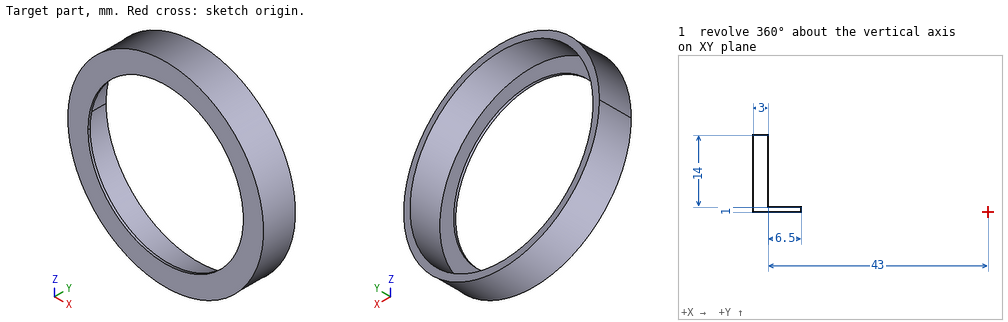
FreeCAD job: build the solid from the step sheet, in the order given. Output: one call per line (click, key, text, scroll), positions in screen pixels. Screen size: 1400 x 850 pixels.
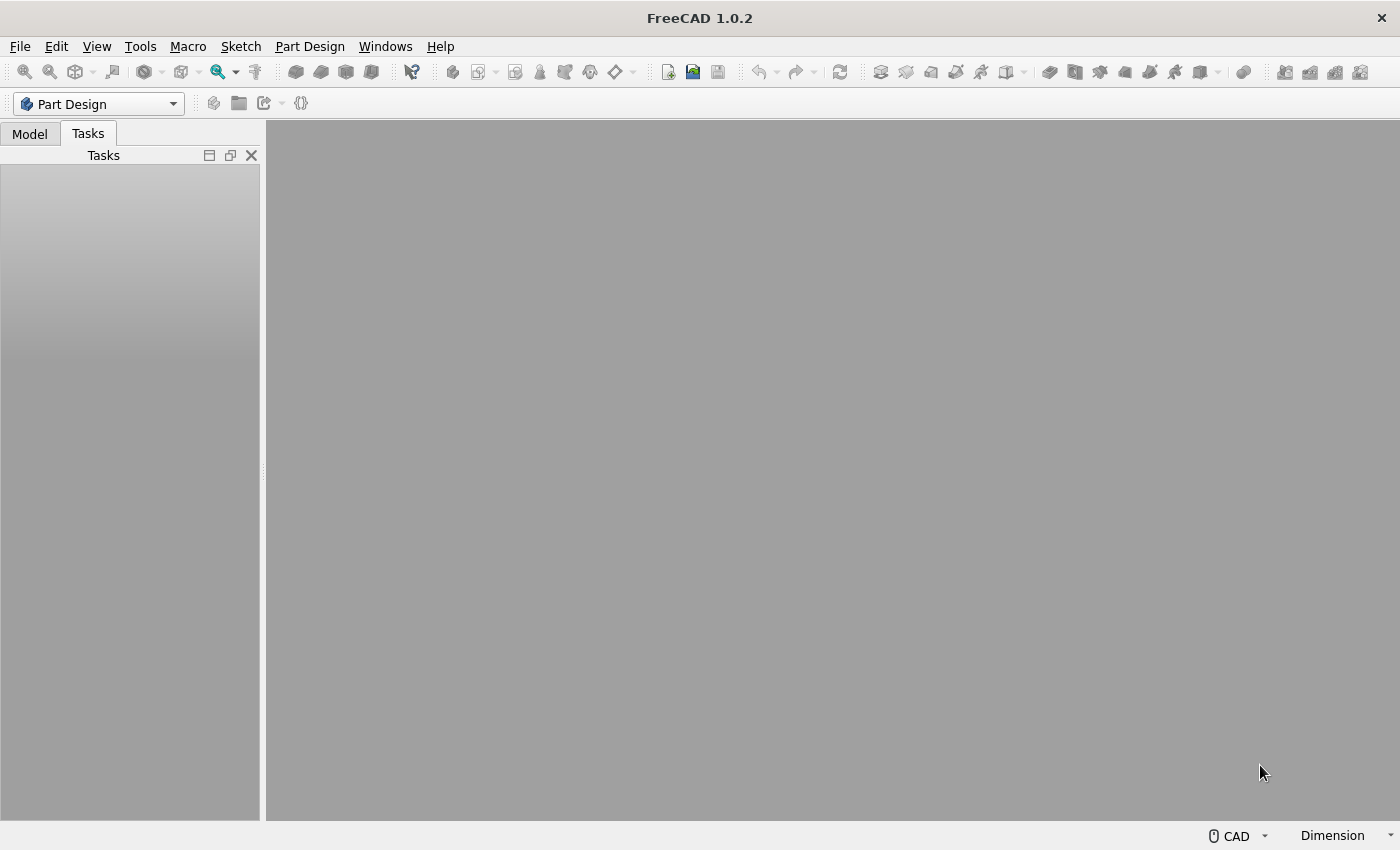
key(ctrl+n)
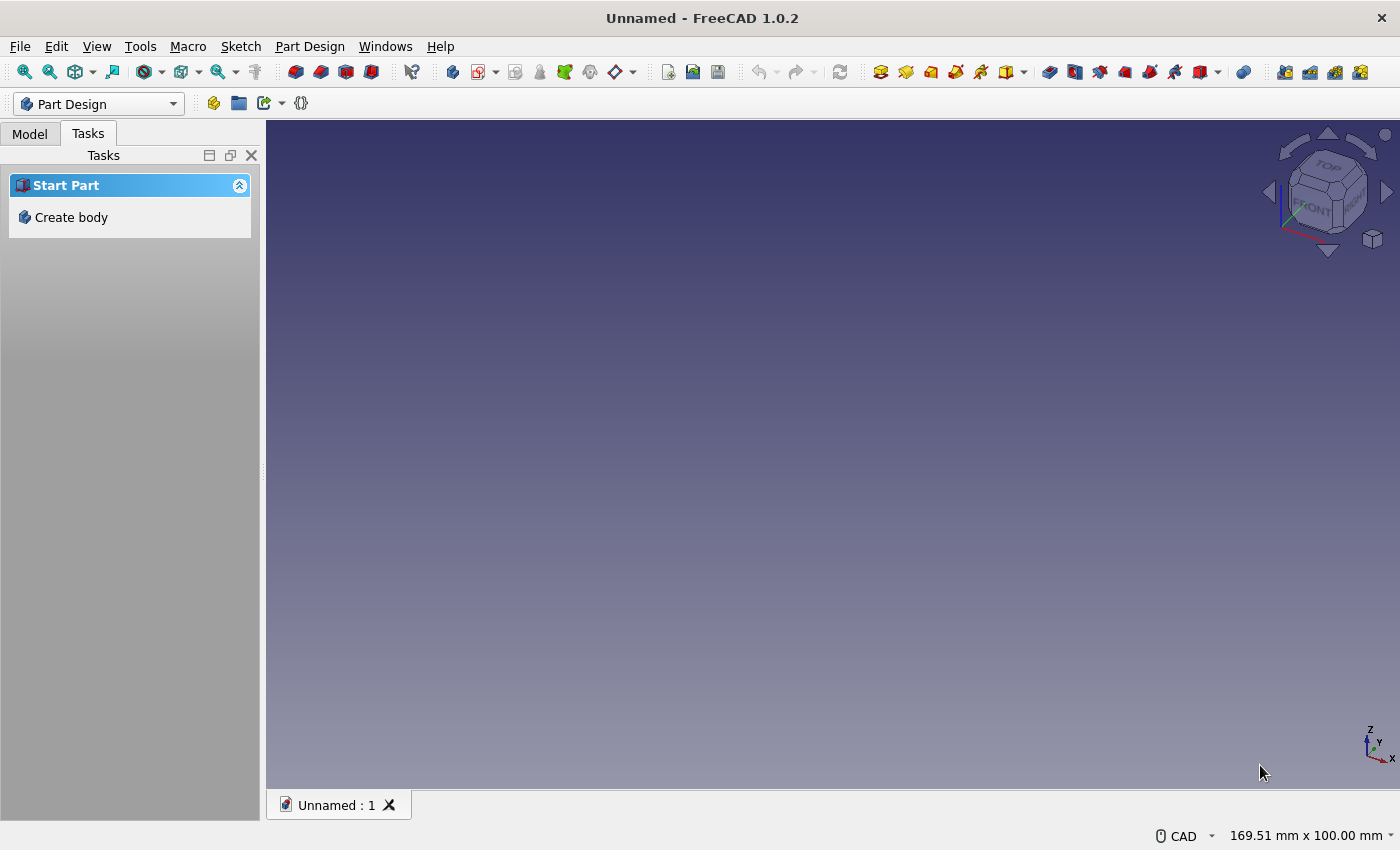
click(478, 72)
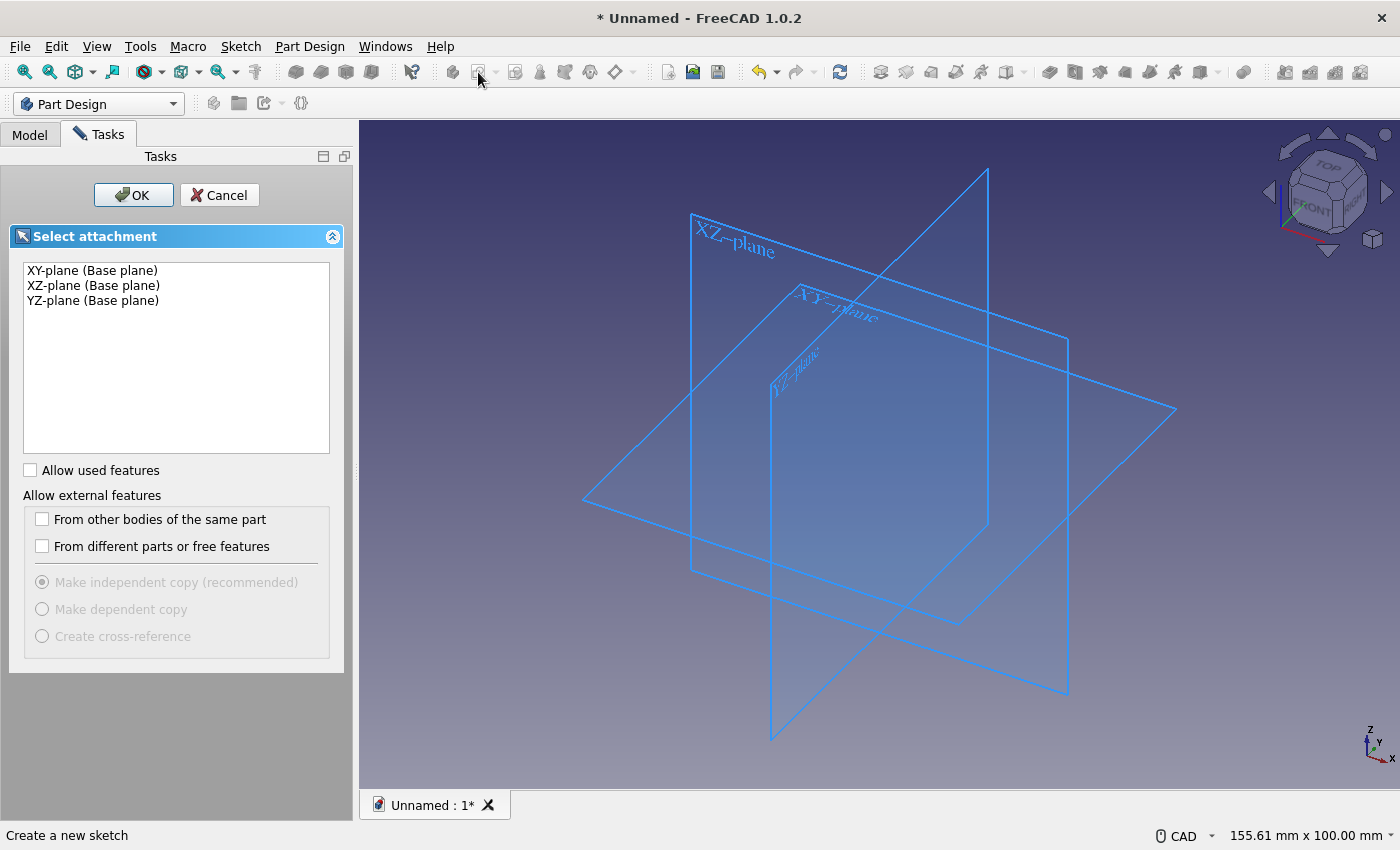
click(84, 270)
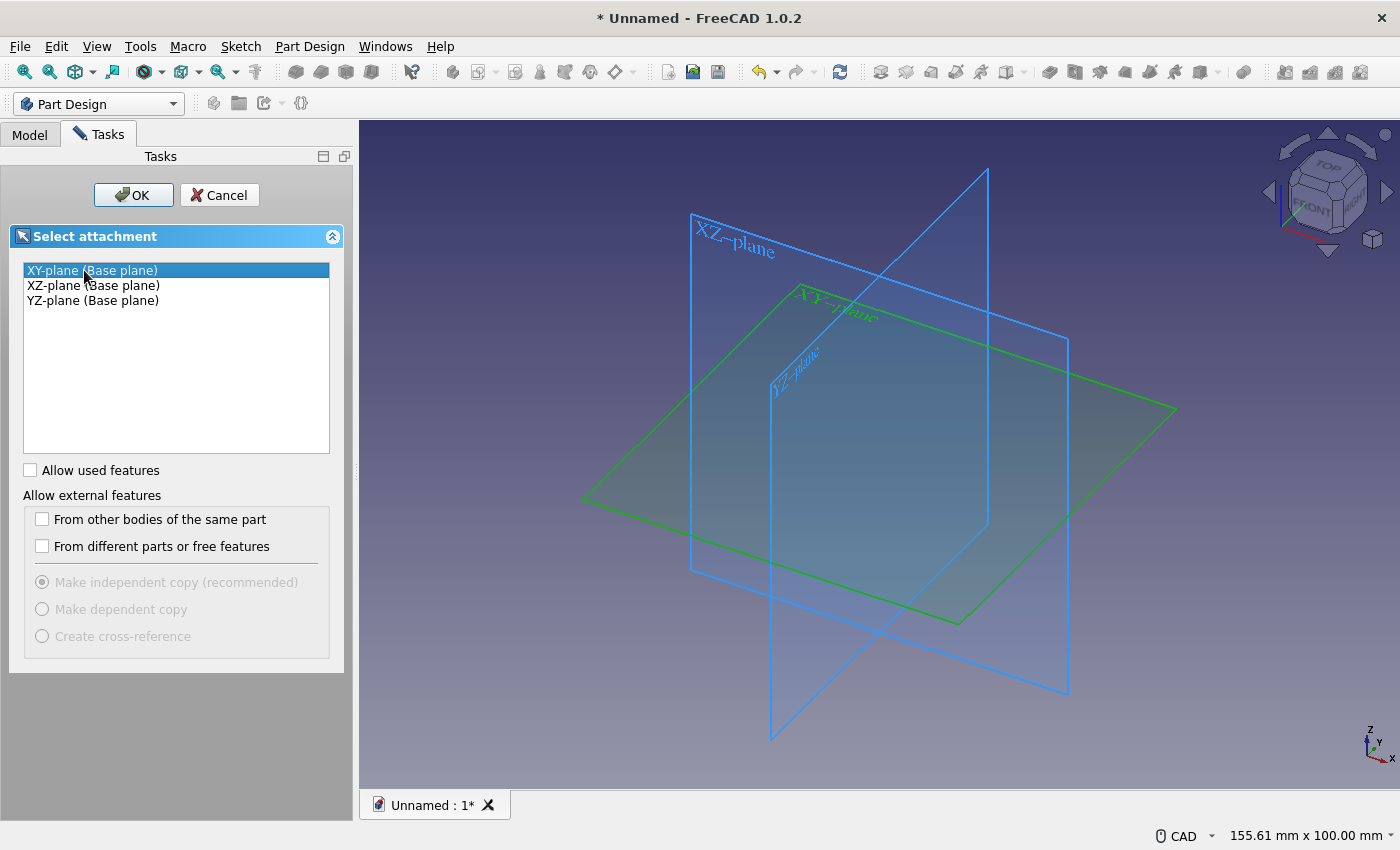
click(134, 195)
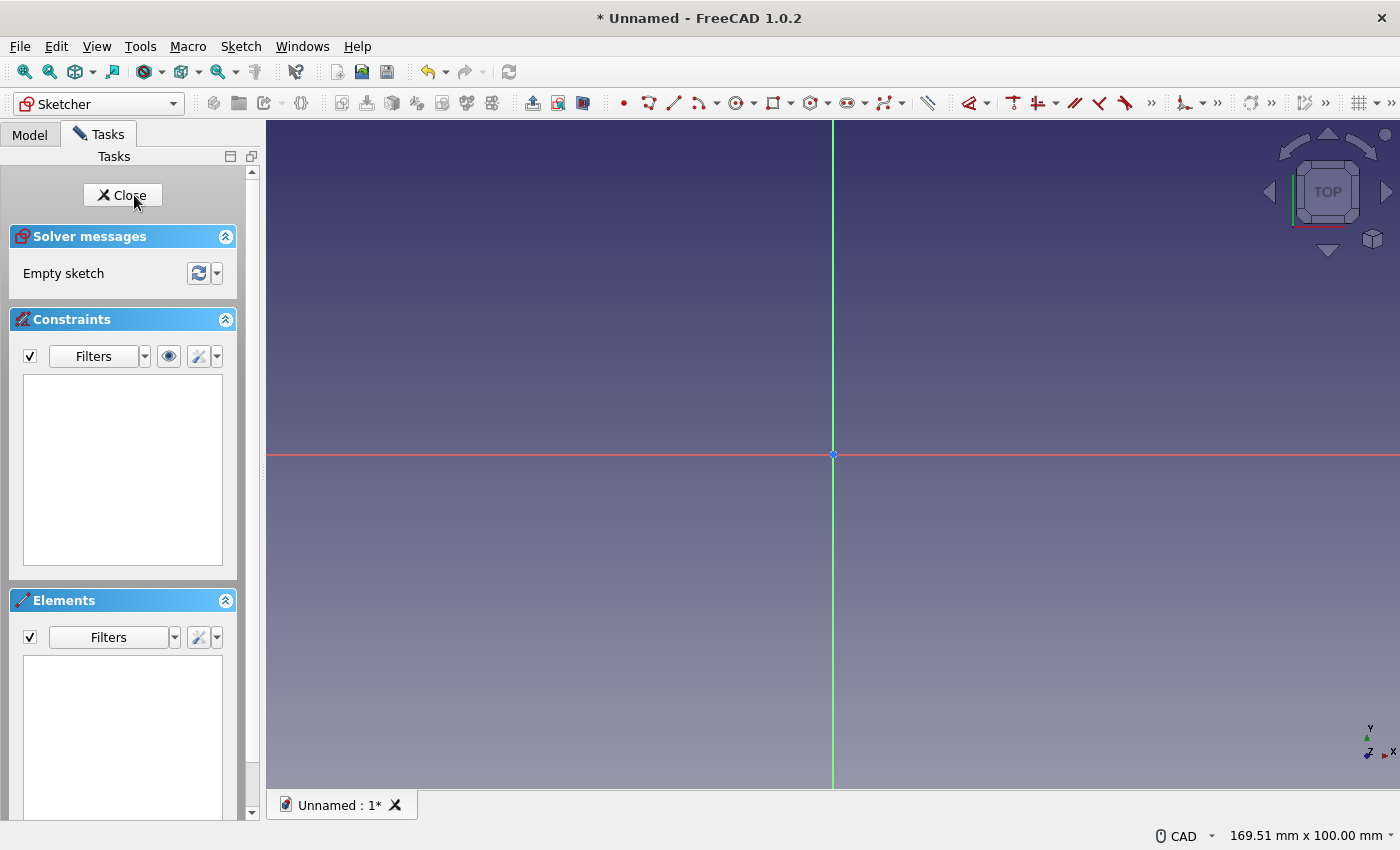
scroll(489, 388, up, 7)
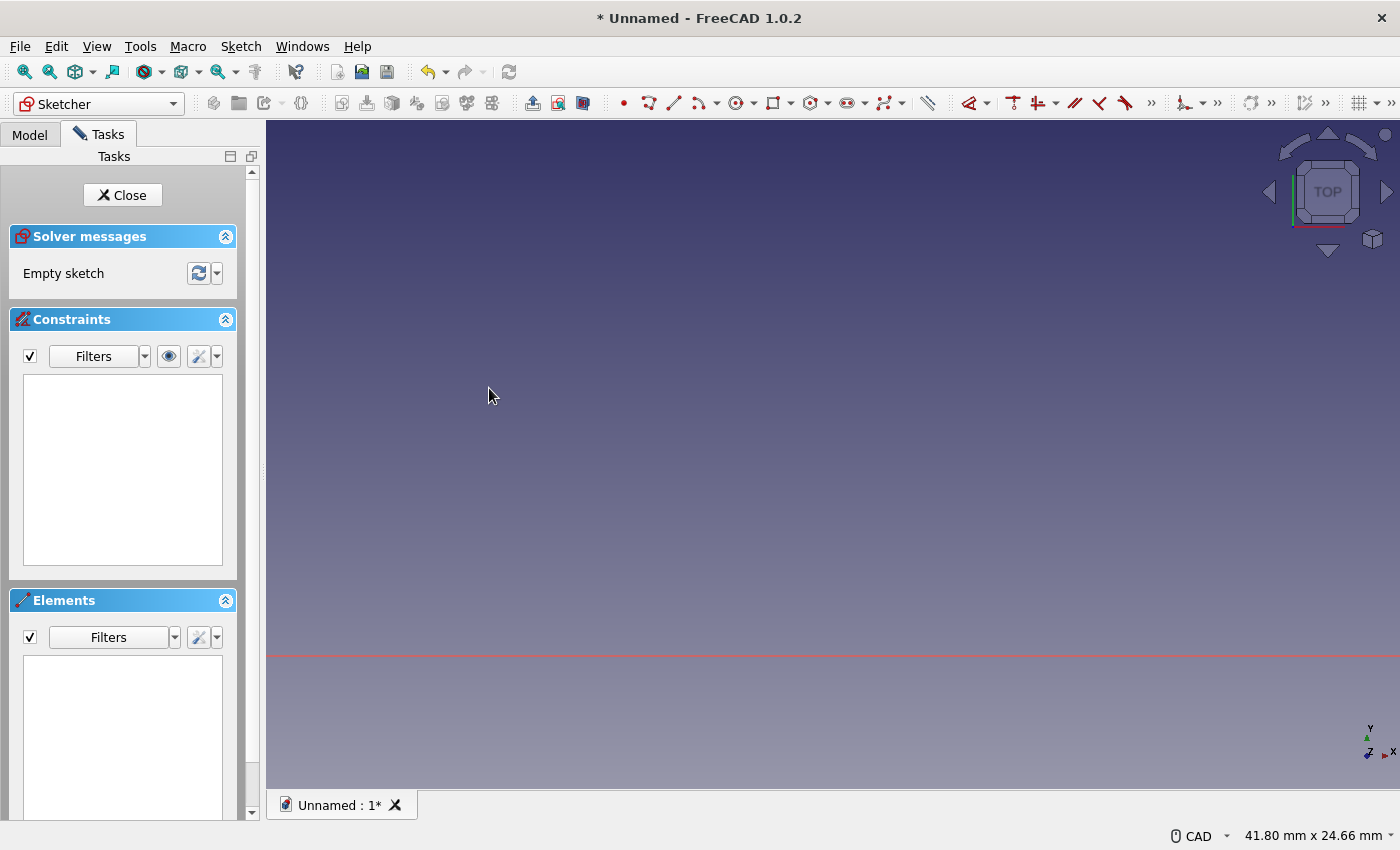
click(649, 104)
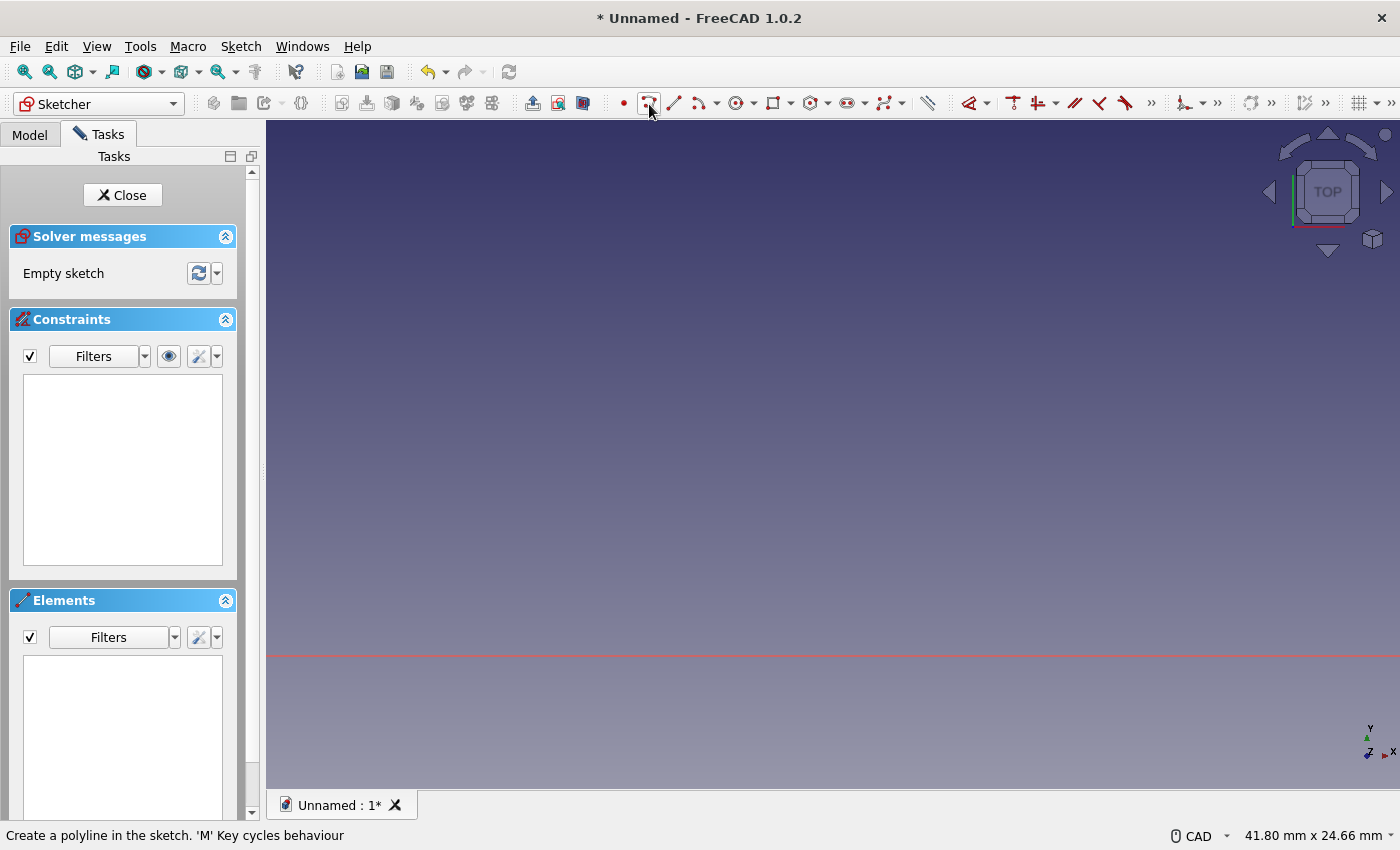
click(893, 656)
click(893, 629)
click(717, 629)
click(717, 250)
click(635, 250)
click(635, 647)
click(893, 656)
key(Escape)
key(Escape)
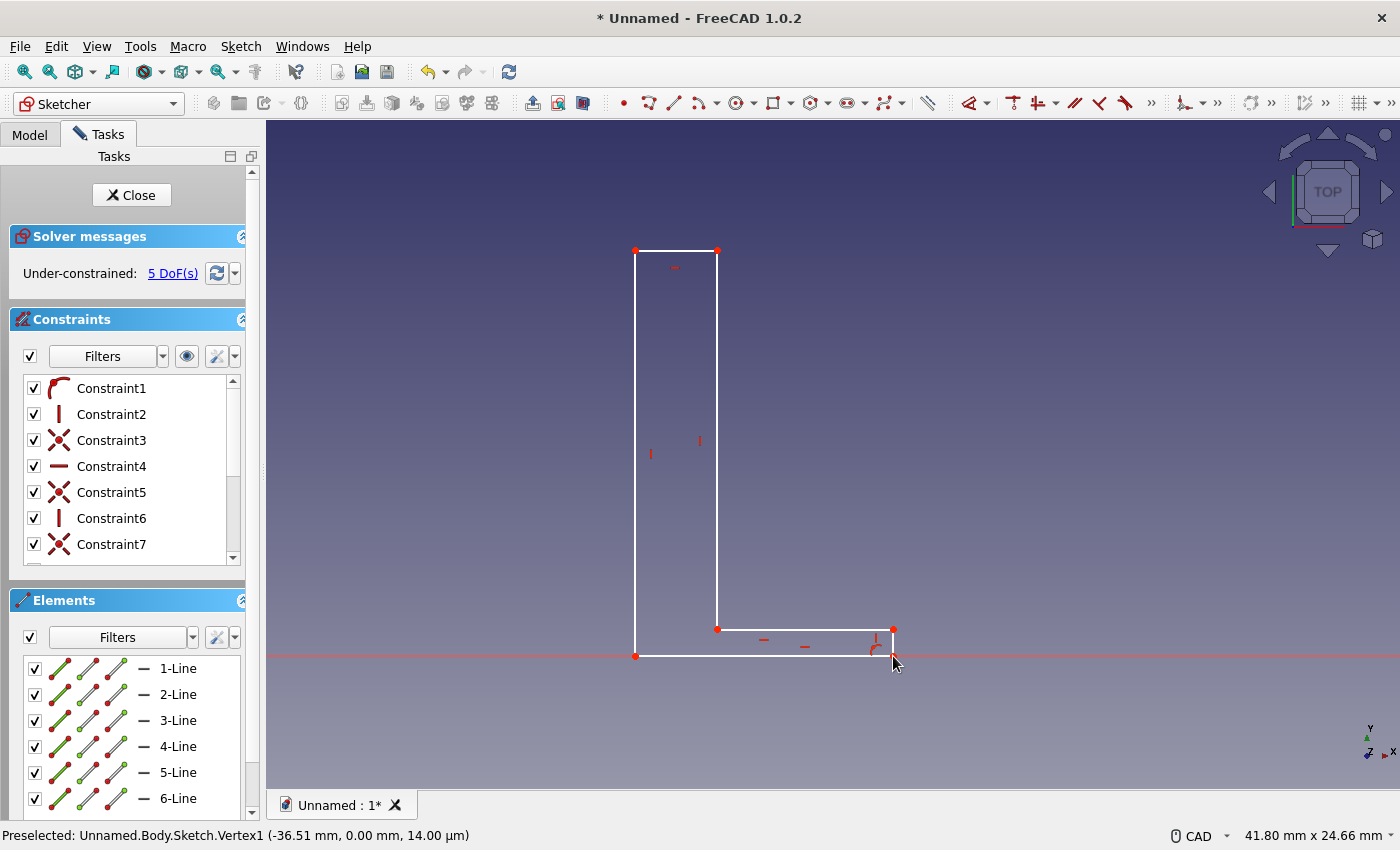
click(968, 104)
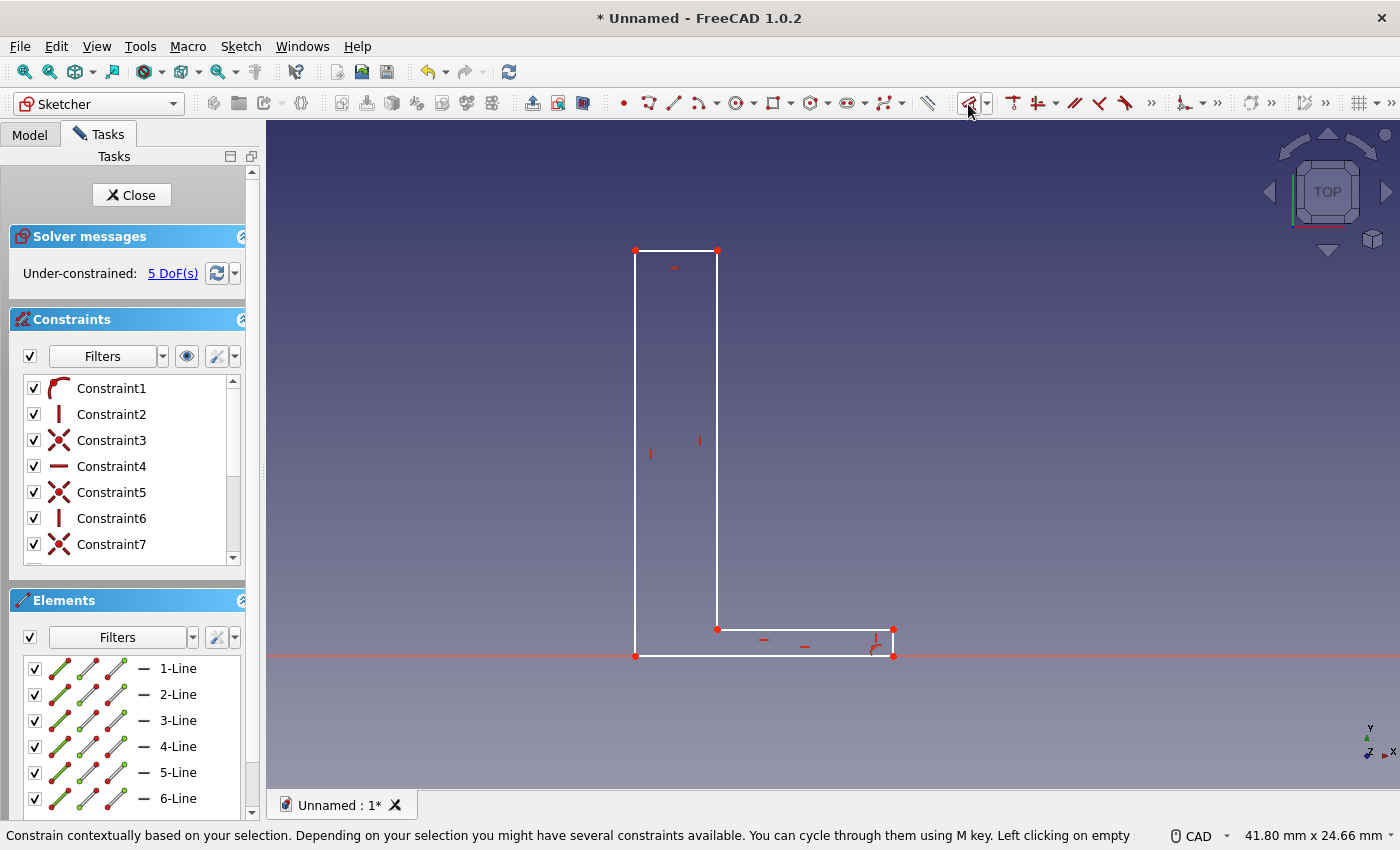
scroll(893, 646, up, 2)